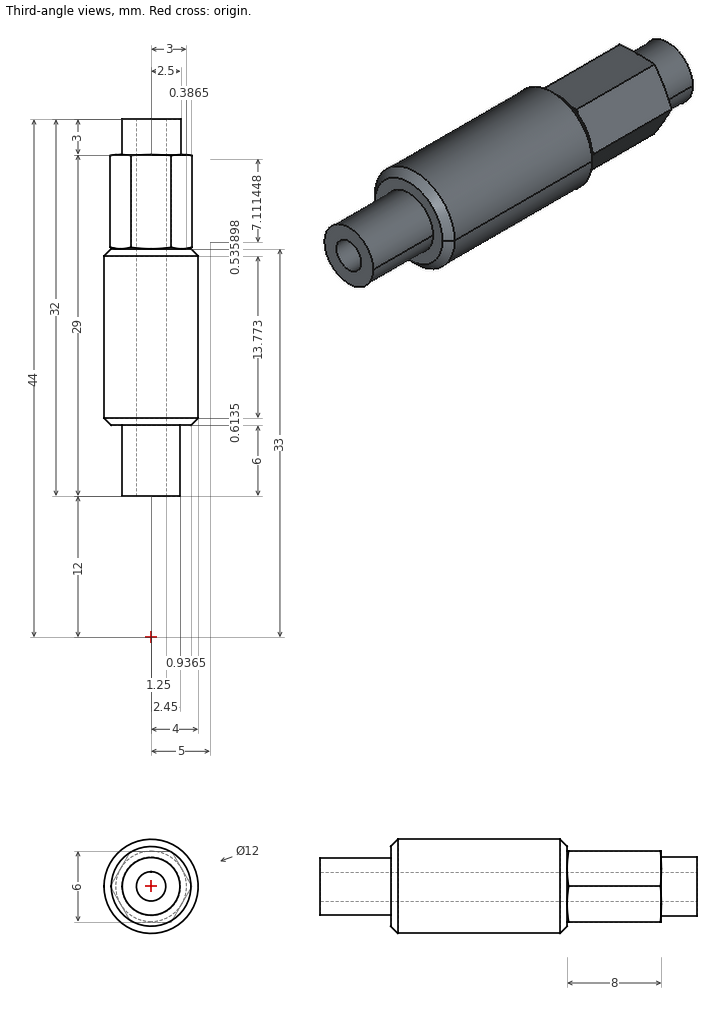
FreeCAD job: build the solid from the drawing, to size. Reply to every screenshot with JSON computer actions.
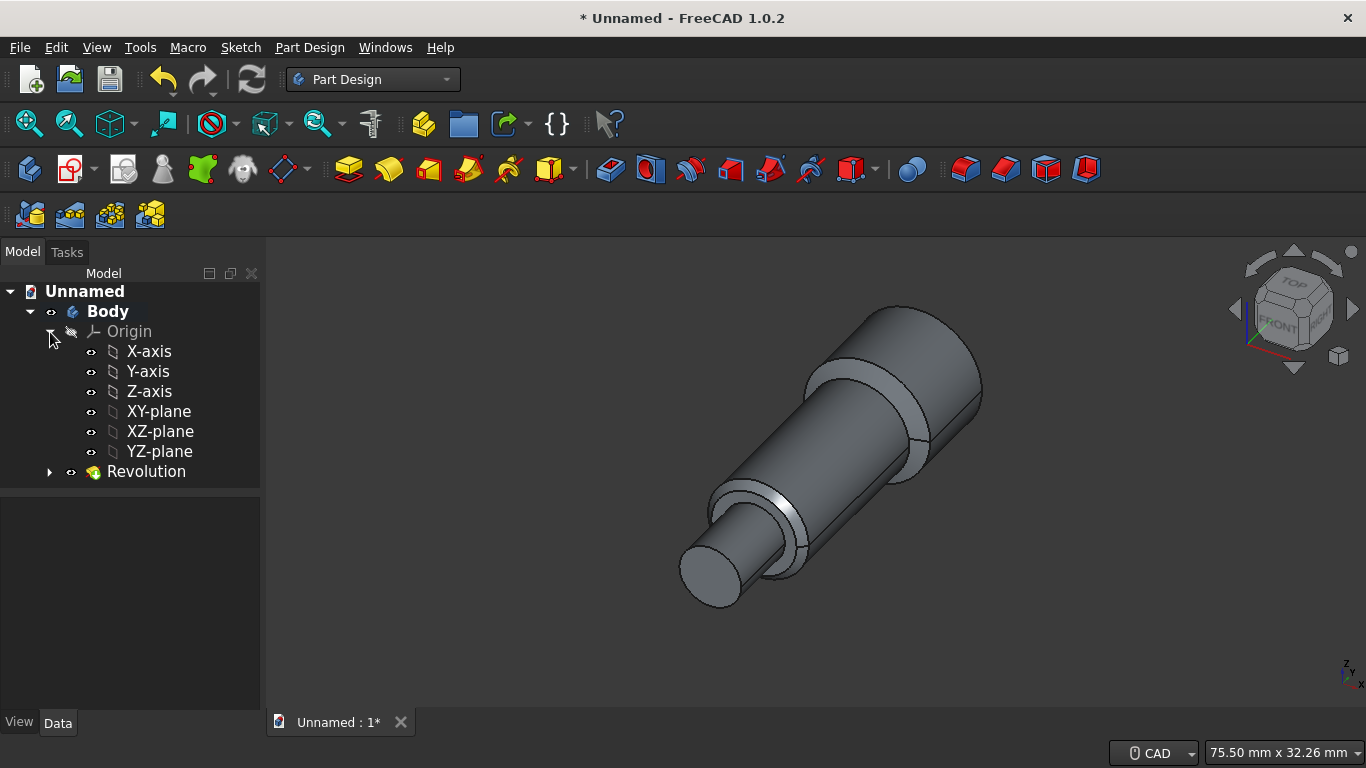
{"action": "left_click", "coordinate": [136, 432]}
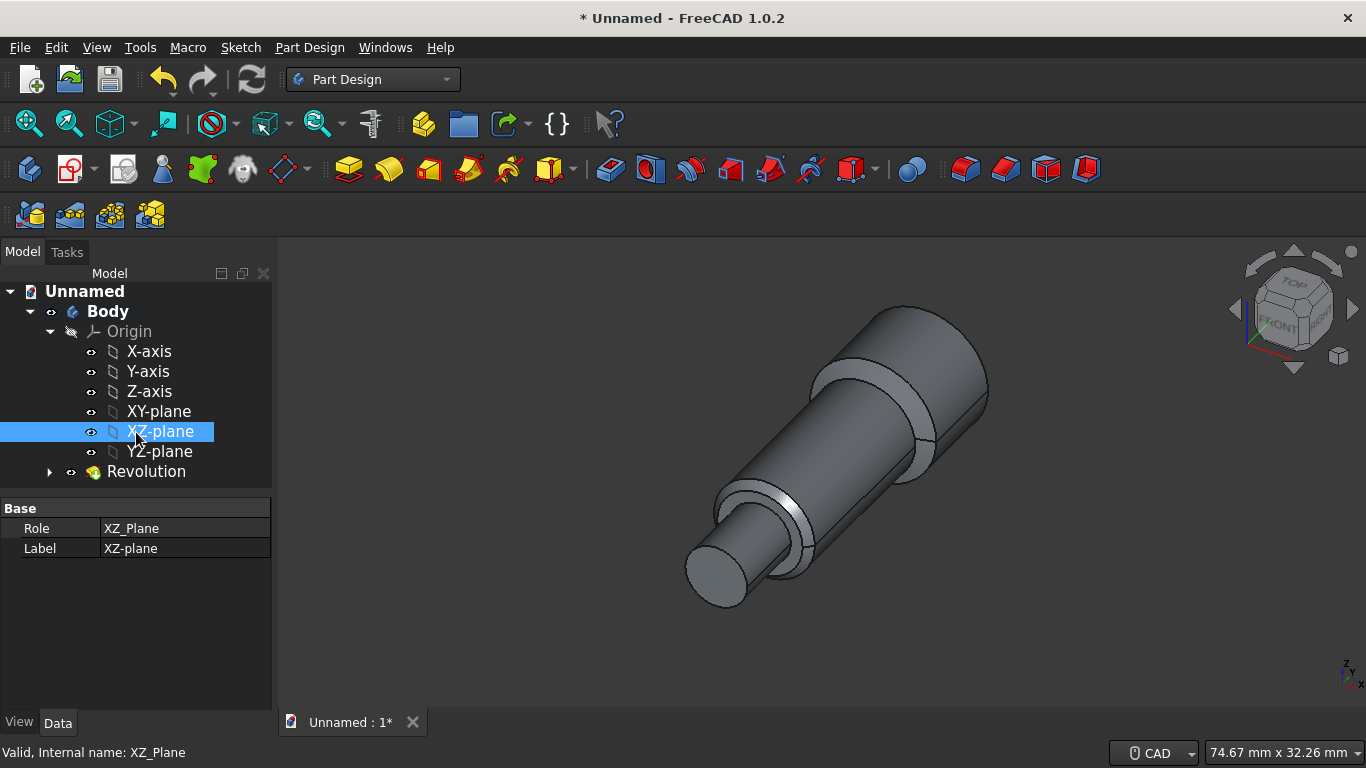
{"action": "left_click", "coordinate": [284, 170]}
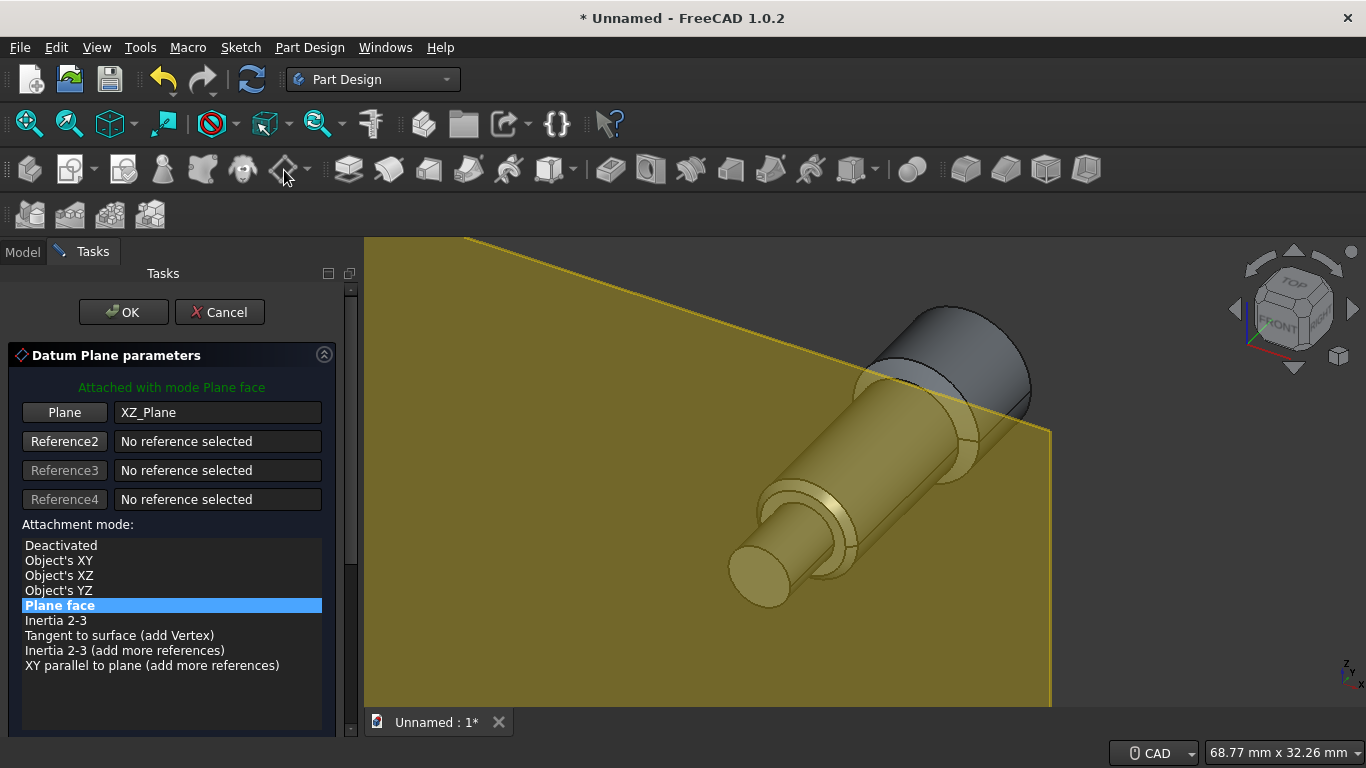
{"action": "scroll", "coordinate": [351, 510], "scroll_direction": "down", "scroll_amount": 3}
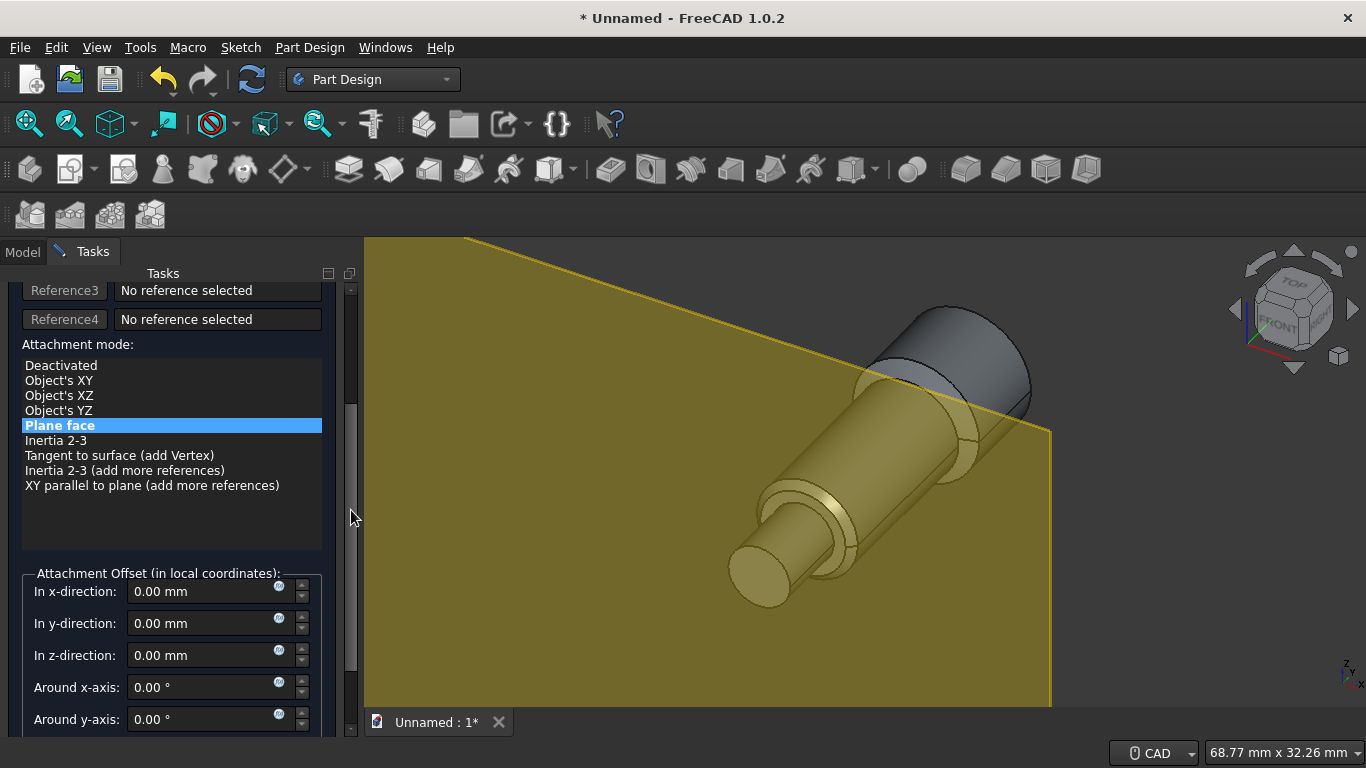
{"action": "triple_click", "coordinate": [210, 655]}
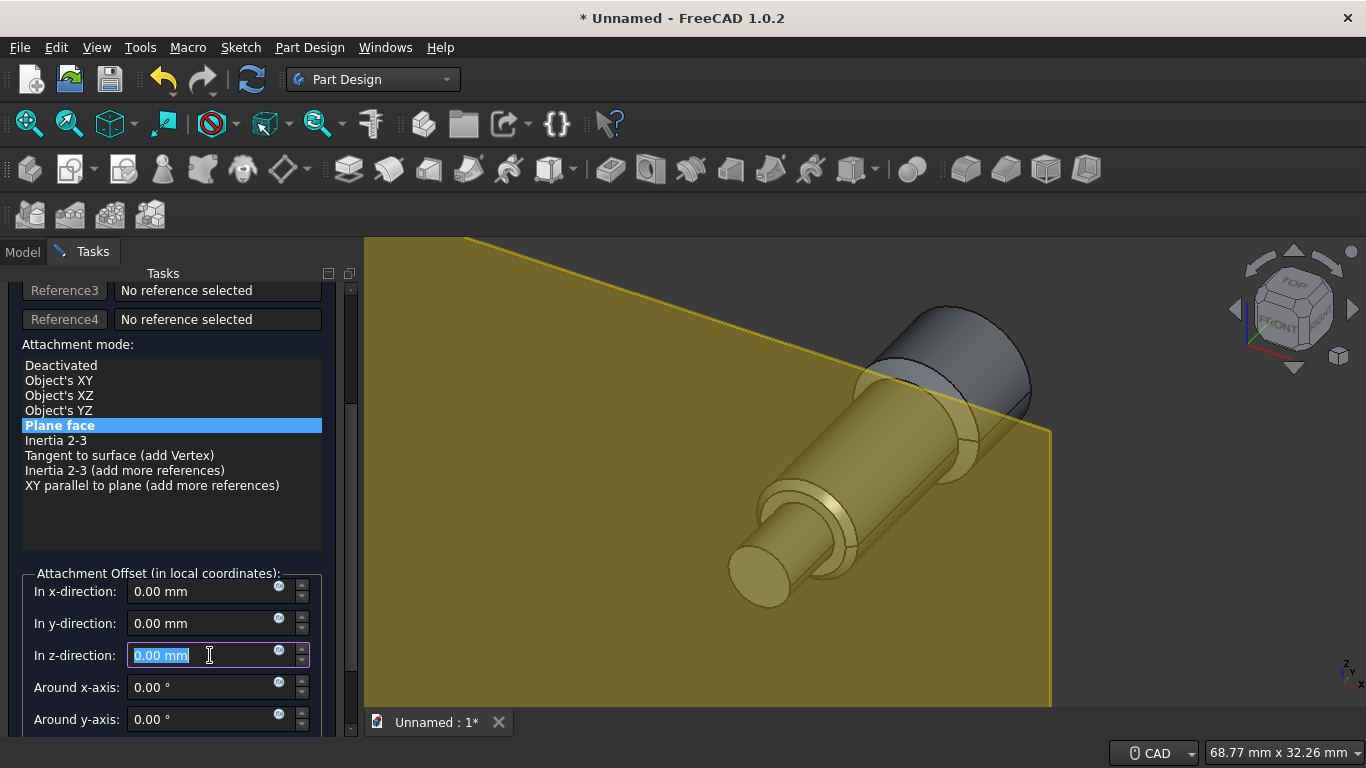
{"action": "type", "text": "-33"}
{"action": "key", "text": "Tab"}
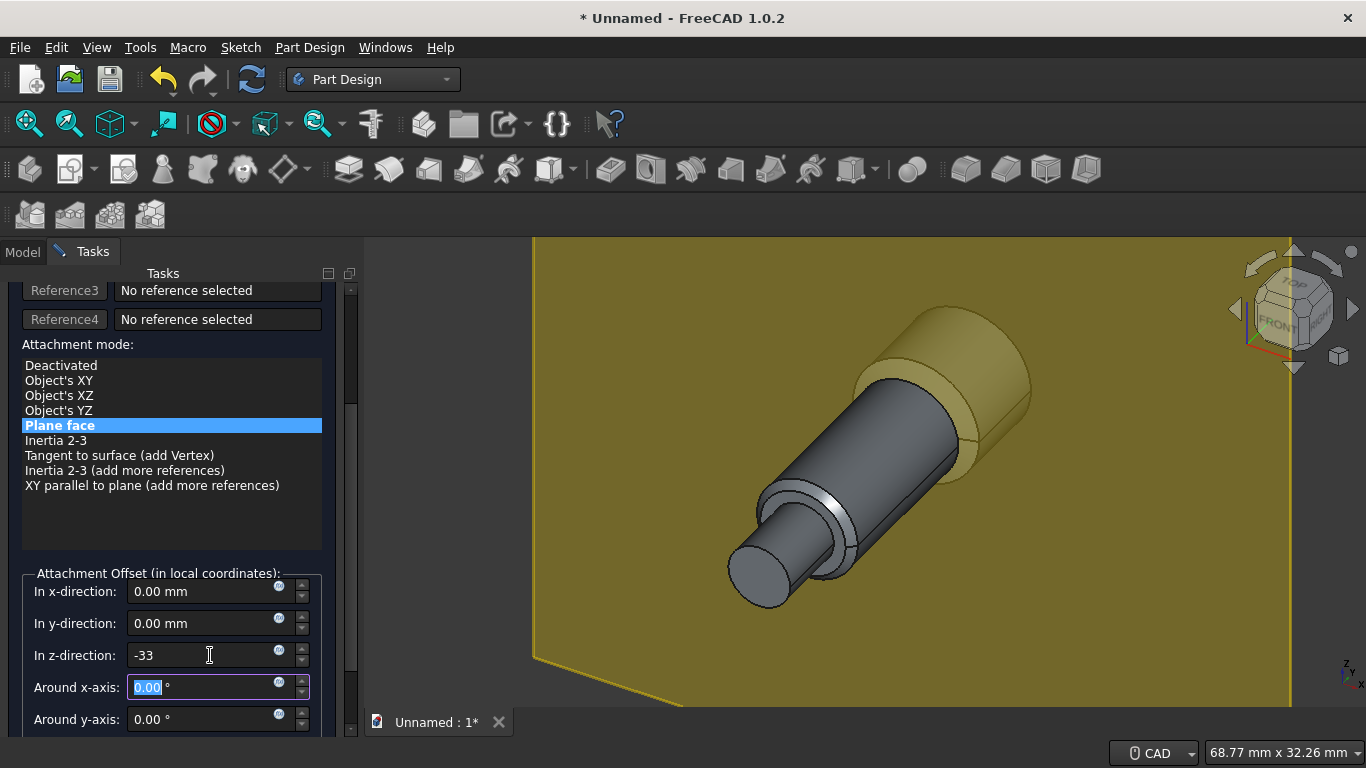
{"action": "scroll", "coordinate": [351, 510], "scroll_direction": "up", "scroll_amount": 4}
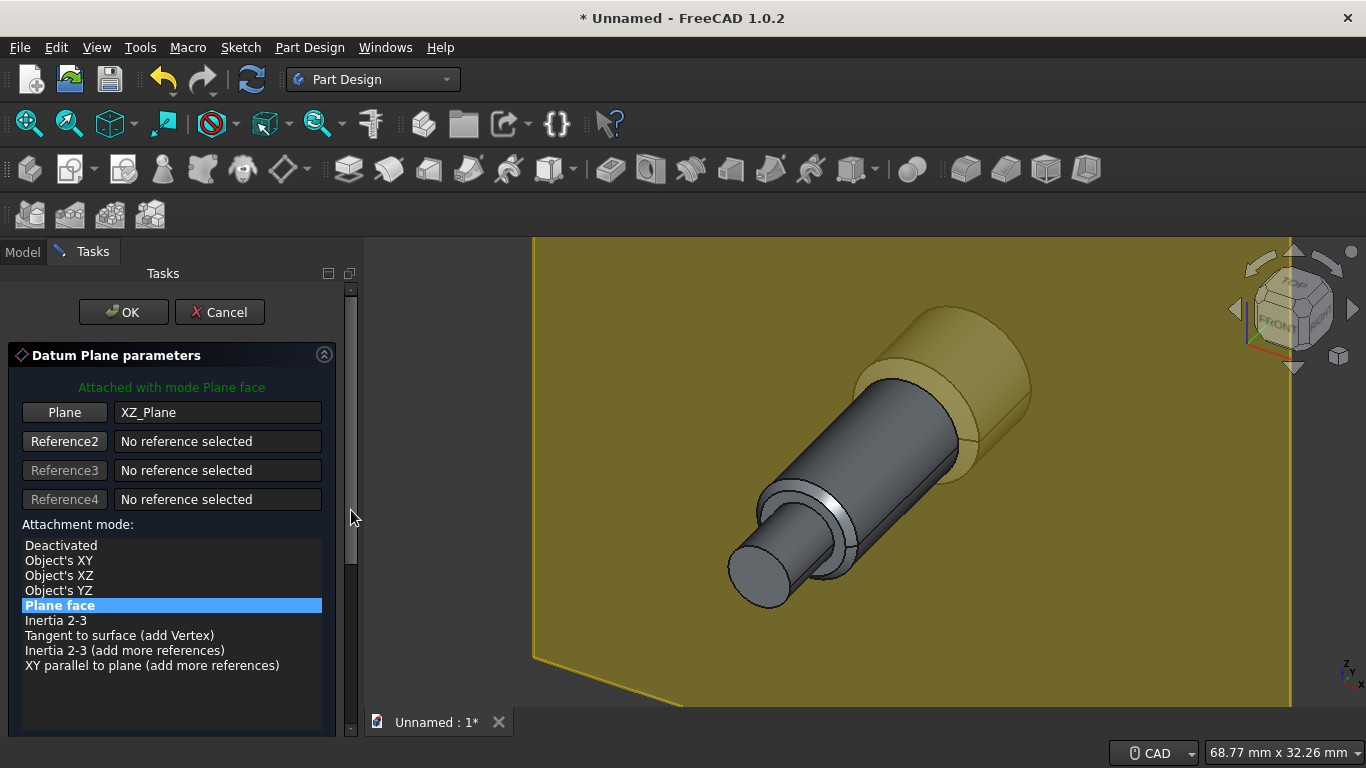
{"action": "left_click", "coordinate": [124, 312]}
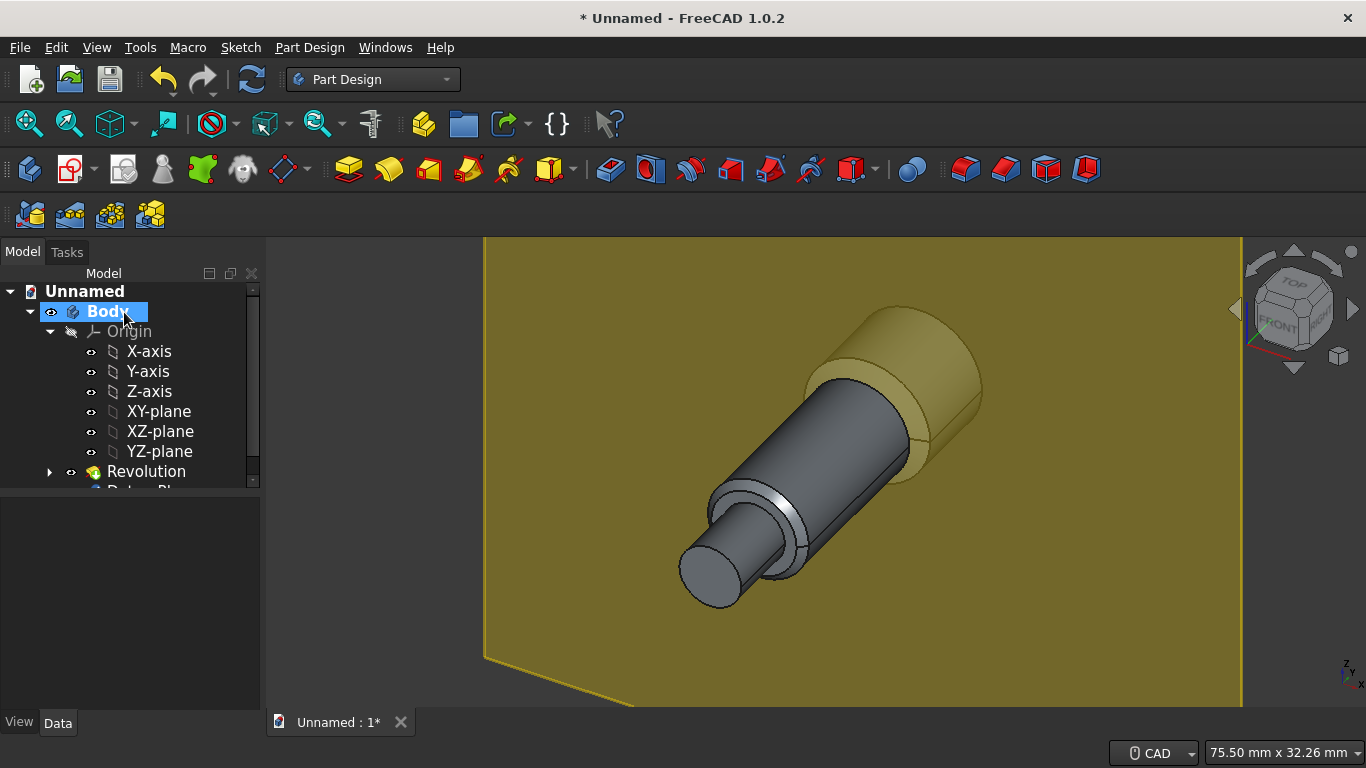
{"action": "scroll", "coordinate": [100, 387], "scroll_direction": "down", "scroll_amount": 3}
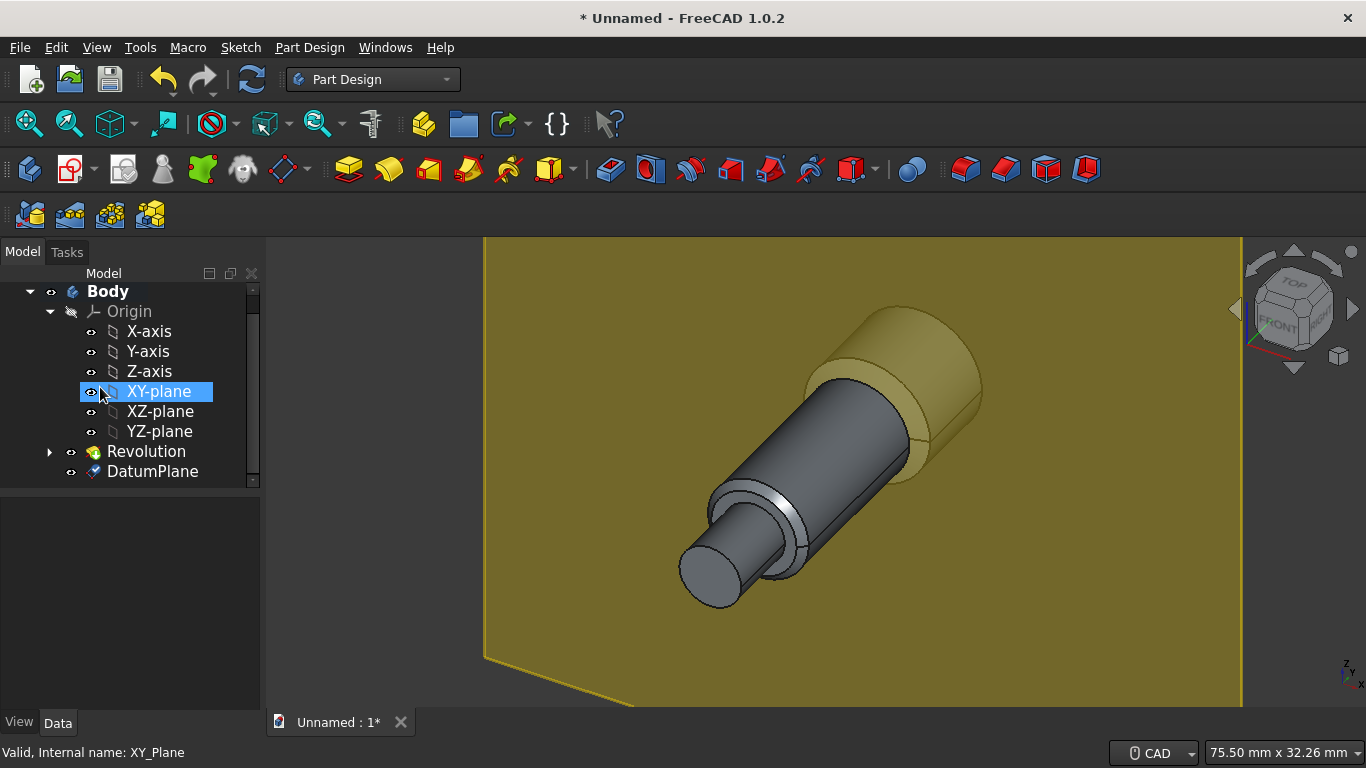
{"action": "left_click", "coordinate": [116, 472]}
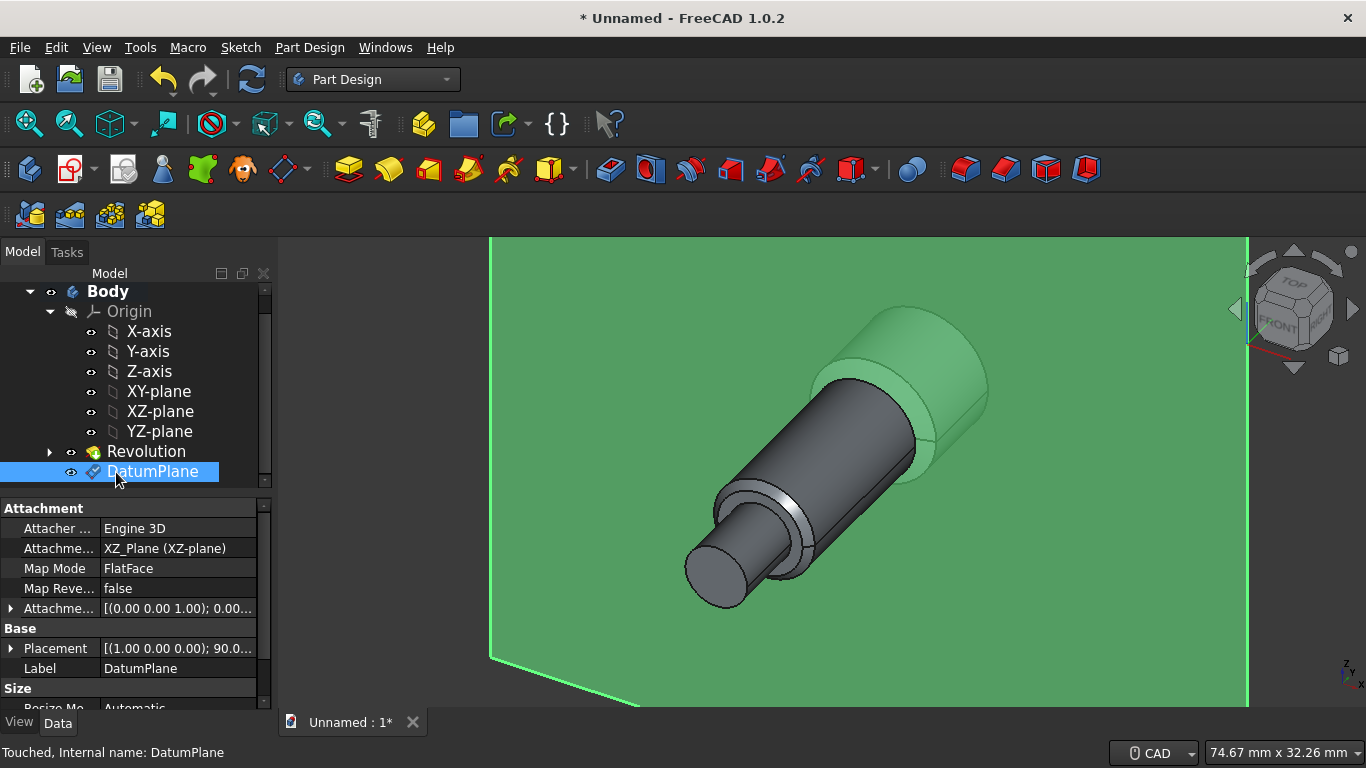
{"action": "left_click", "coordinate": [70, 170]}